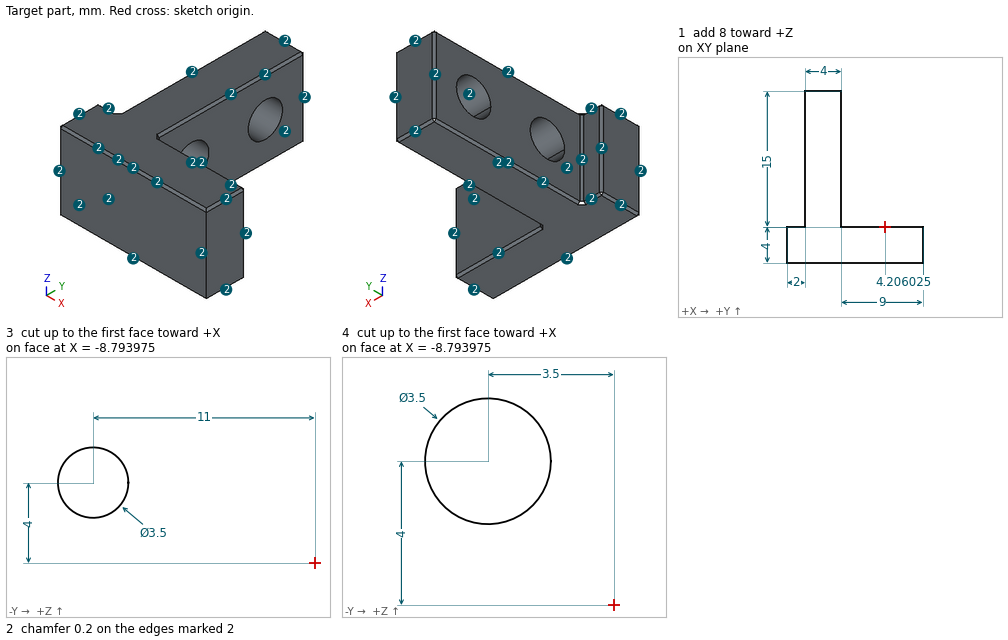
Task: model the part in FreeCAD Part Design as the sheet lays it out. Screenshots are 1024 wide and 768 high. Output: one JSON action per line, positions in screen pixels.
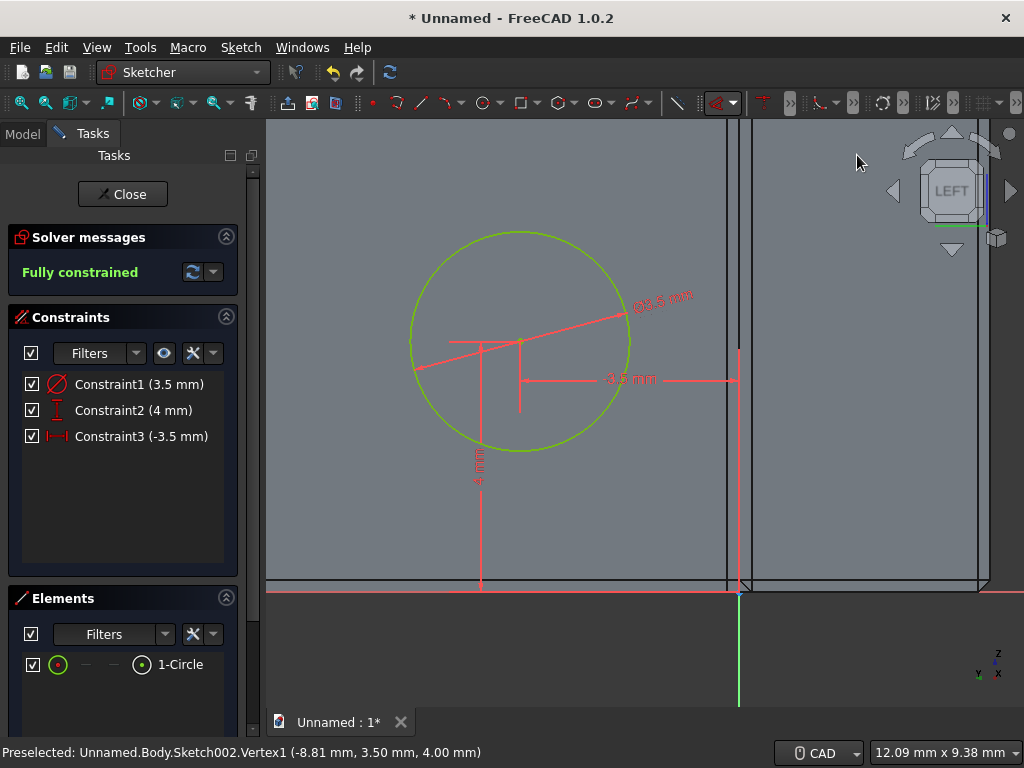
{"action": "left_click", "coordinate": [123, 194]}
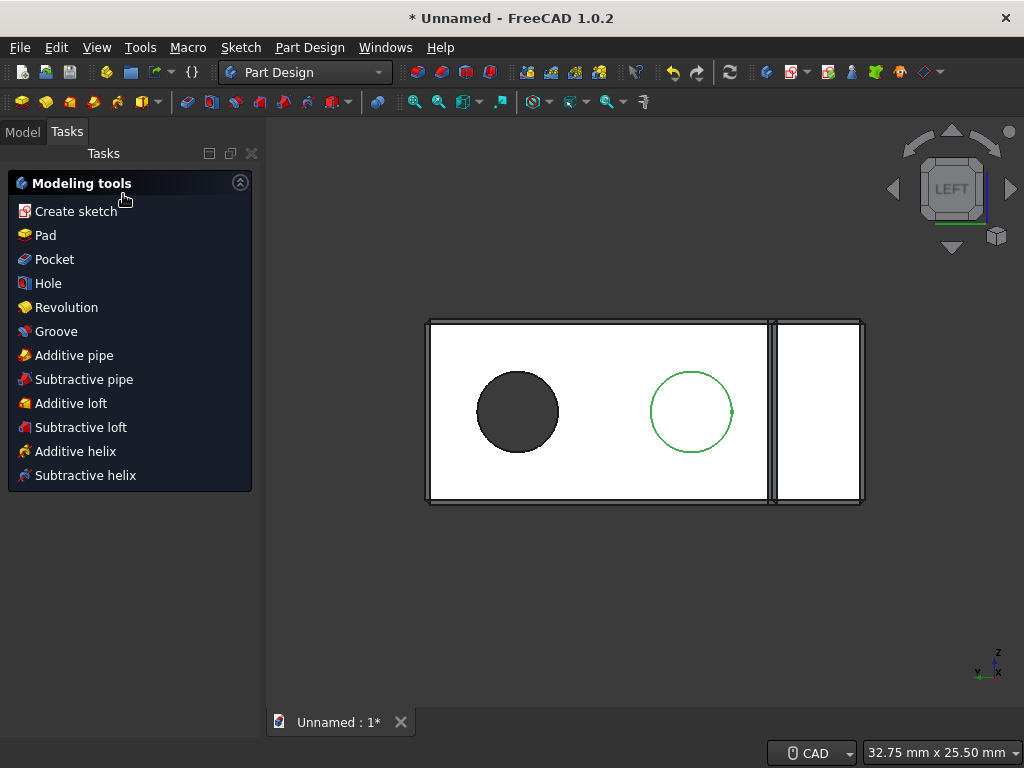
{"action": "left_click", "coordinate": [188, 102]}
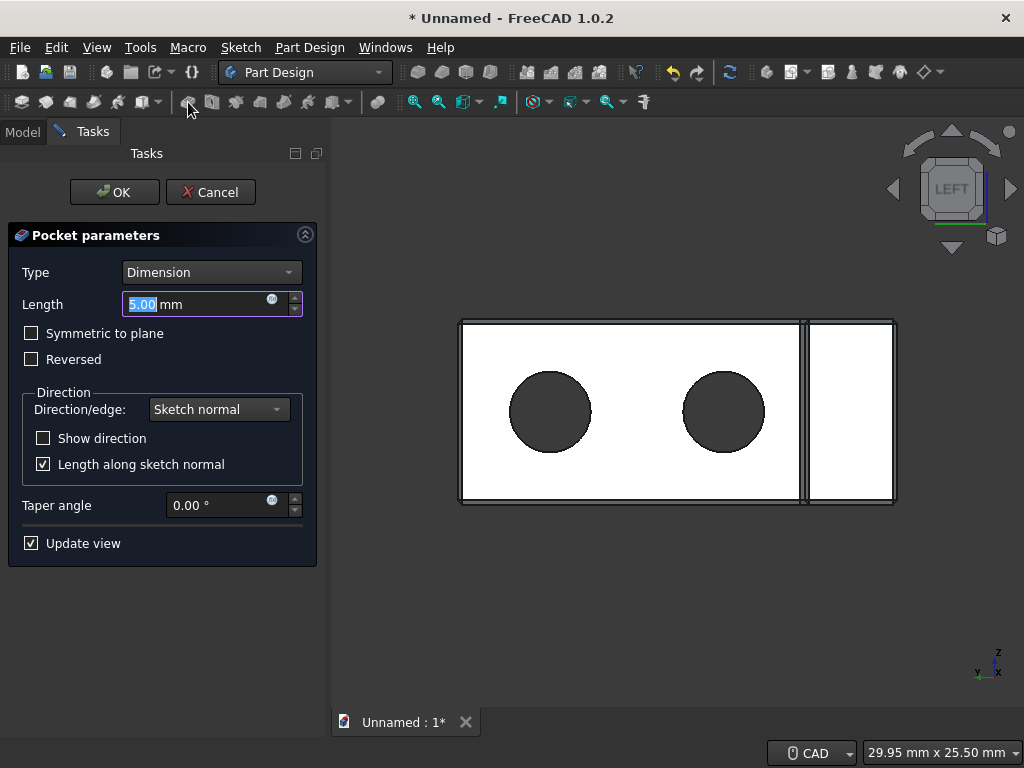
{"action": "left_click", "coordinate": [212, 272]}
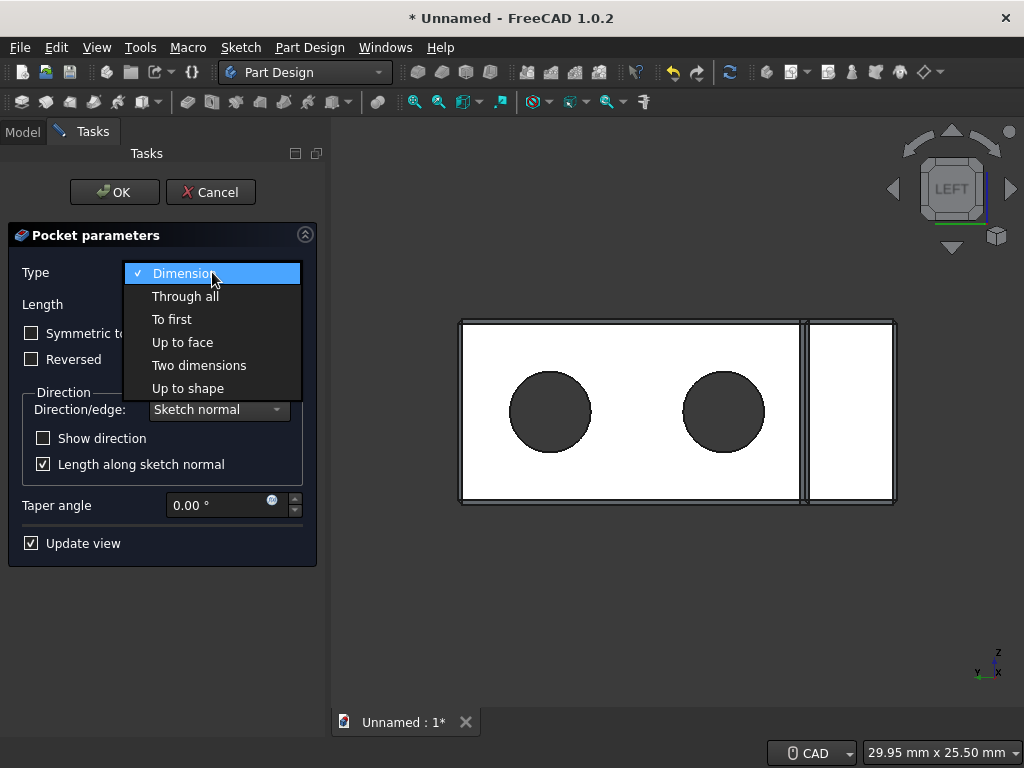
{"action": "left_click", "coordinate": [212, 320]}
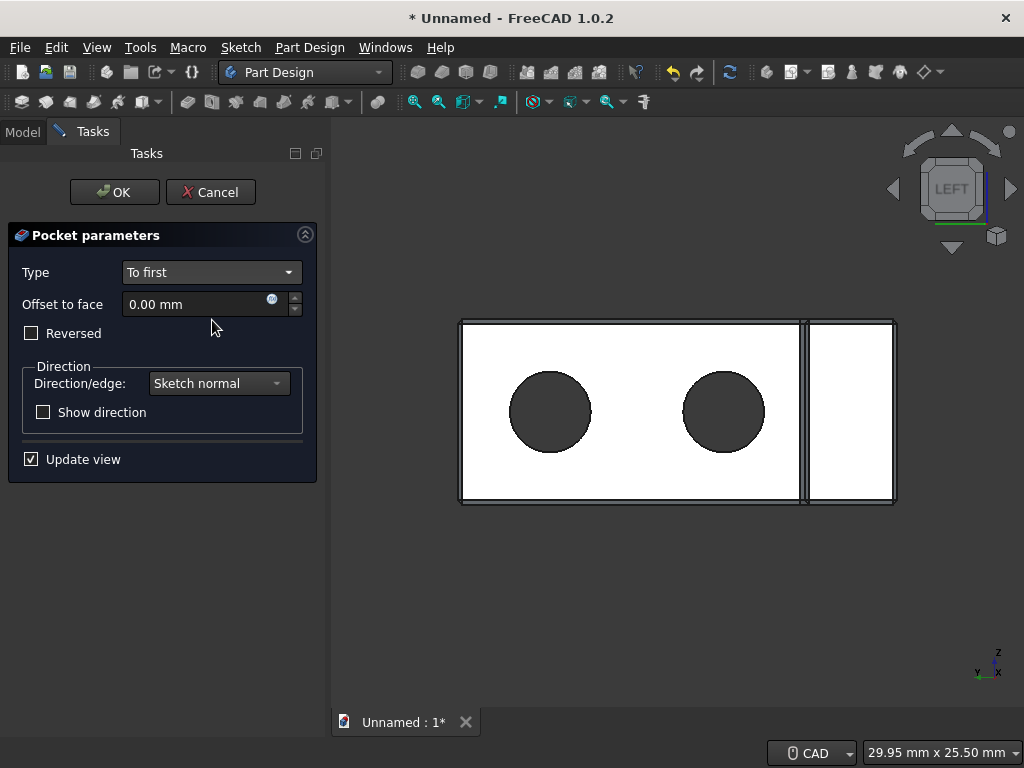
{"action": "left_click", "coordinate": [115, 192]}